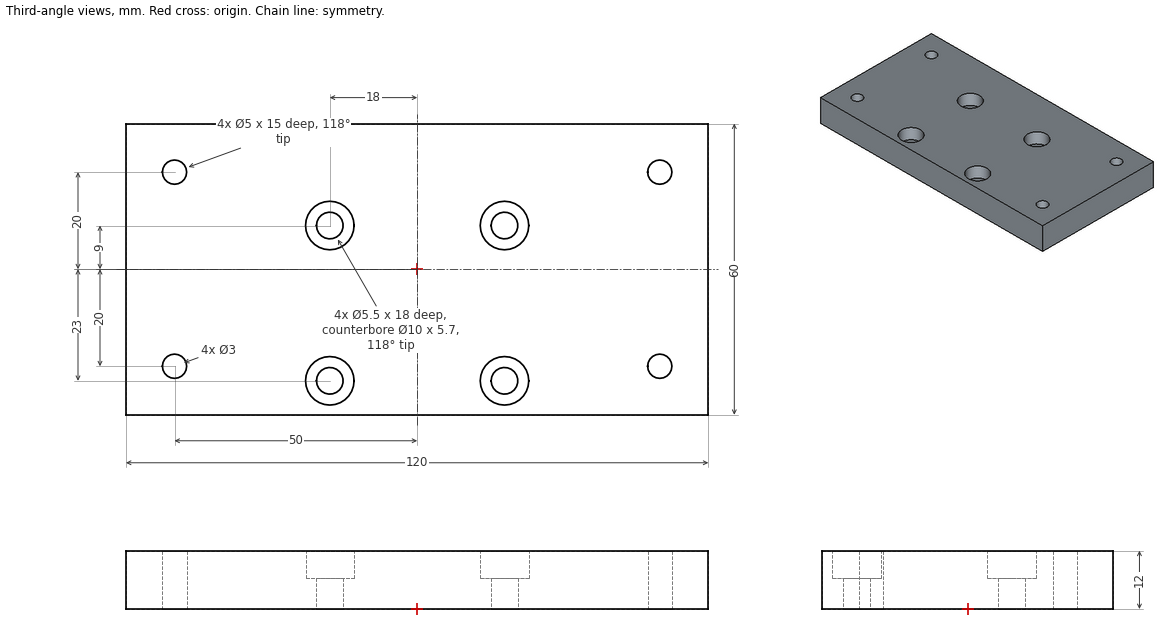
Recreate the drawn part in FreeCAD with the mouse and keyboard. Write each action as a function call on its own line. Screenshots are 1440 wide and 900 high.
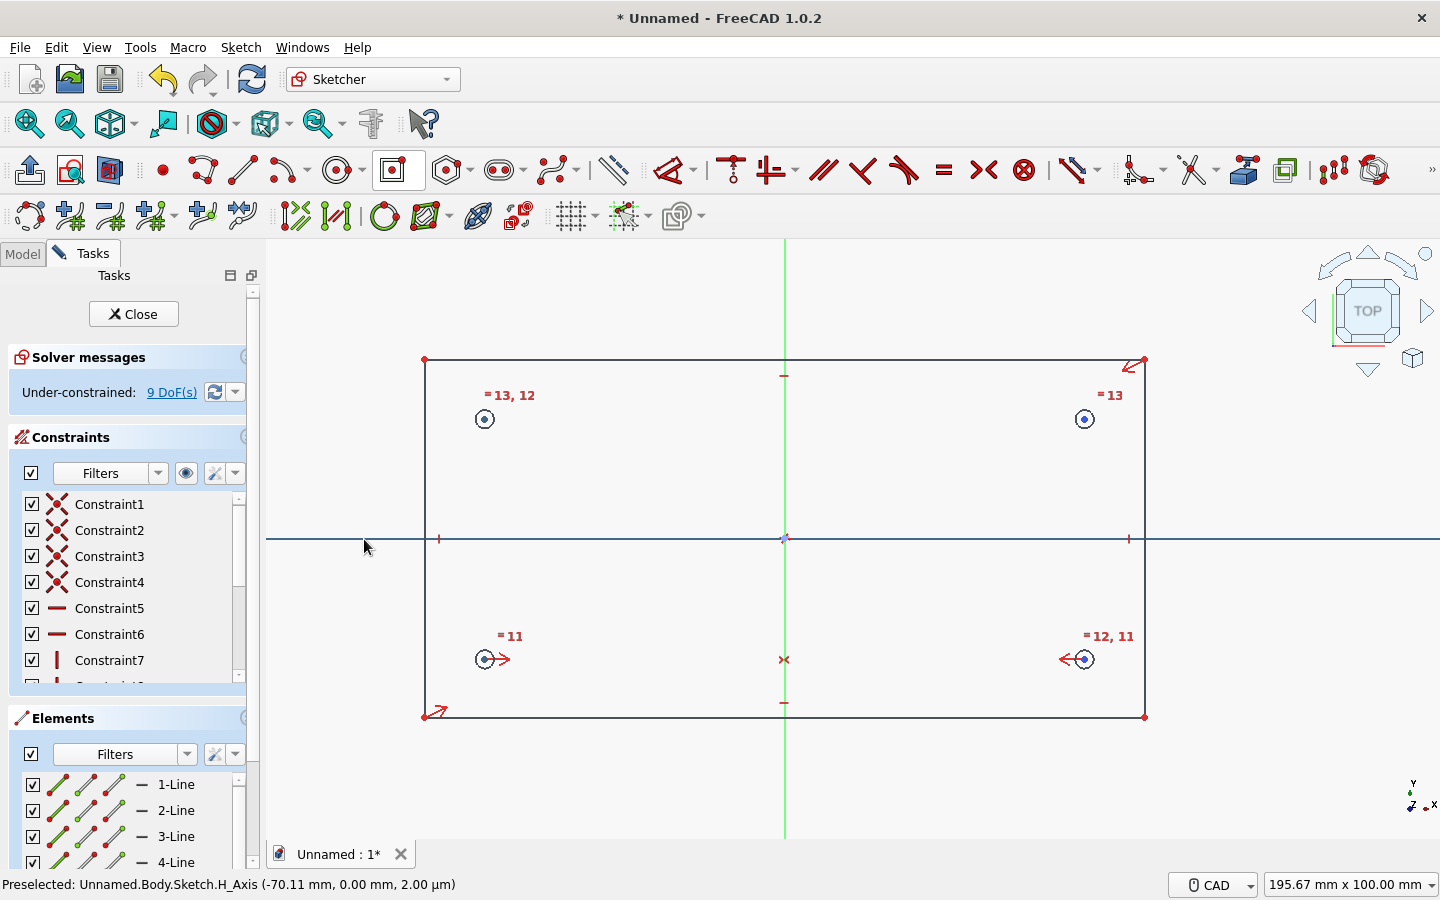
click(984, 170)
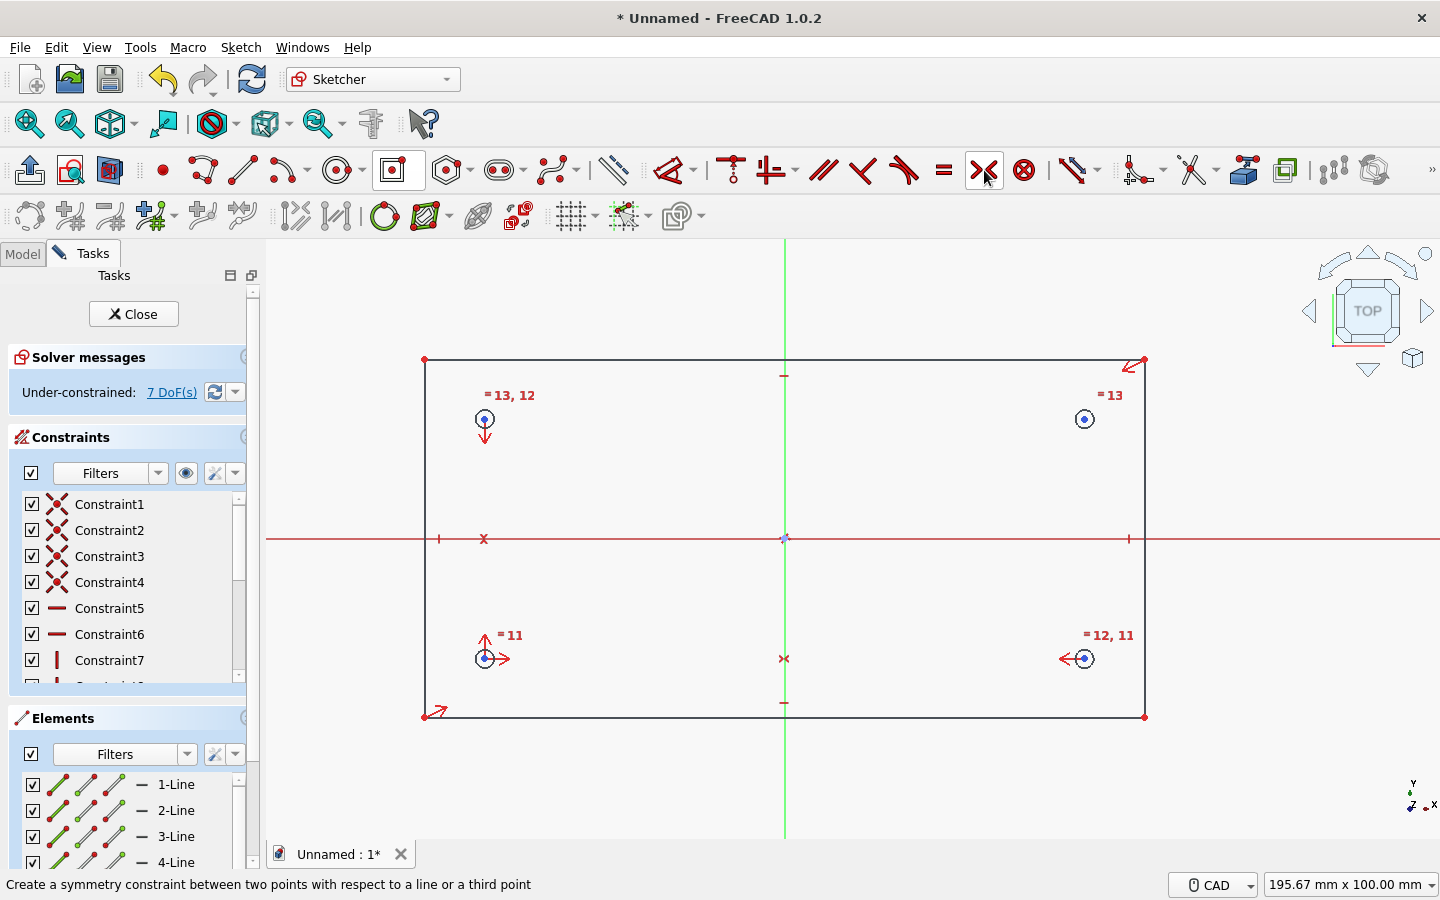
click(1085, 659)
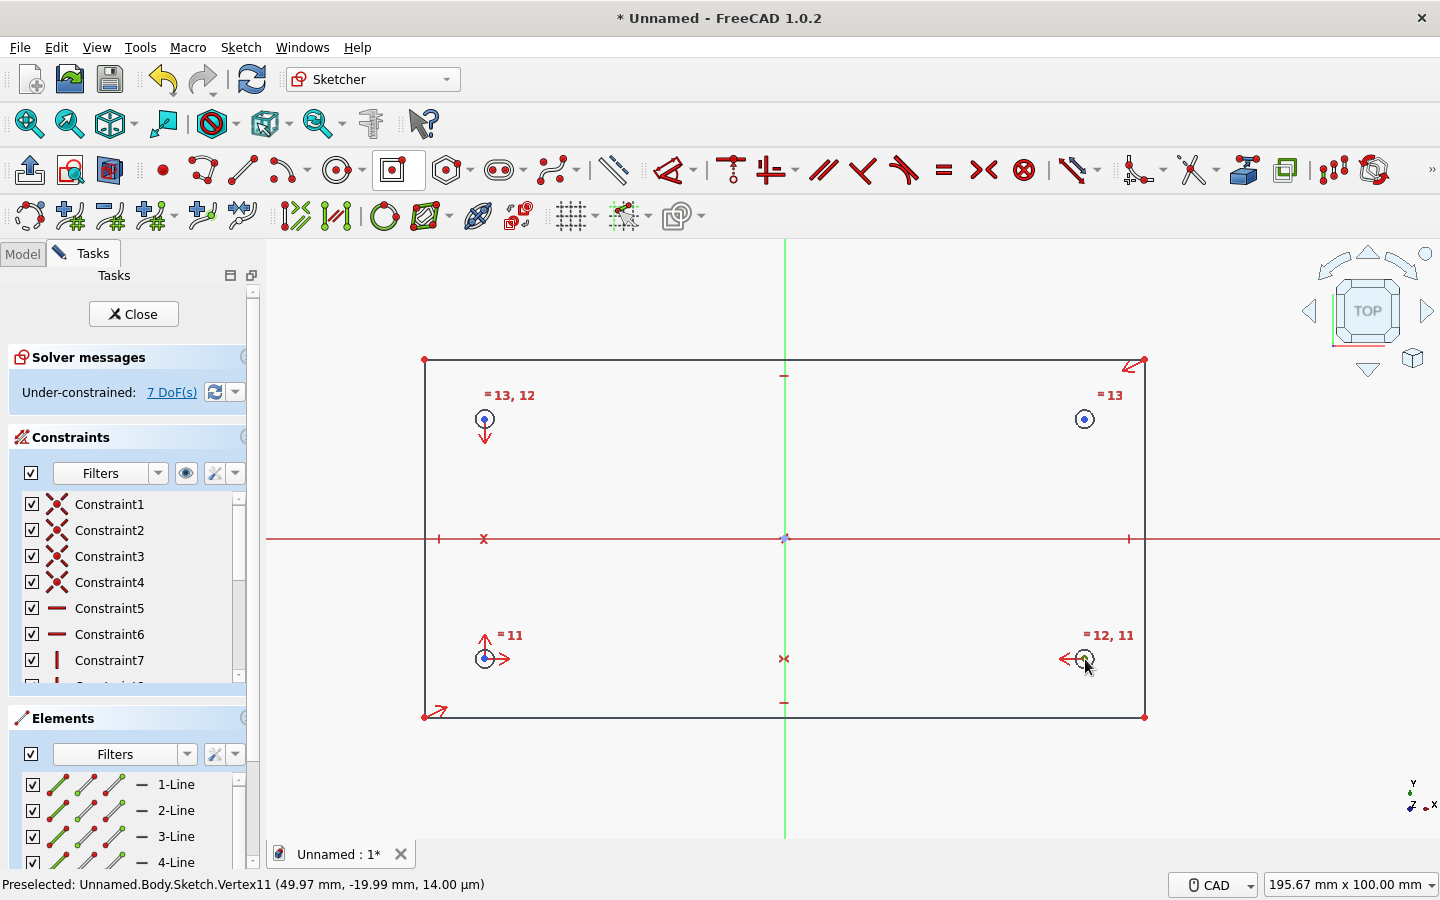
click(1085, 419)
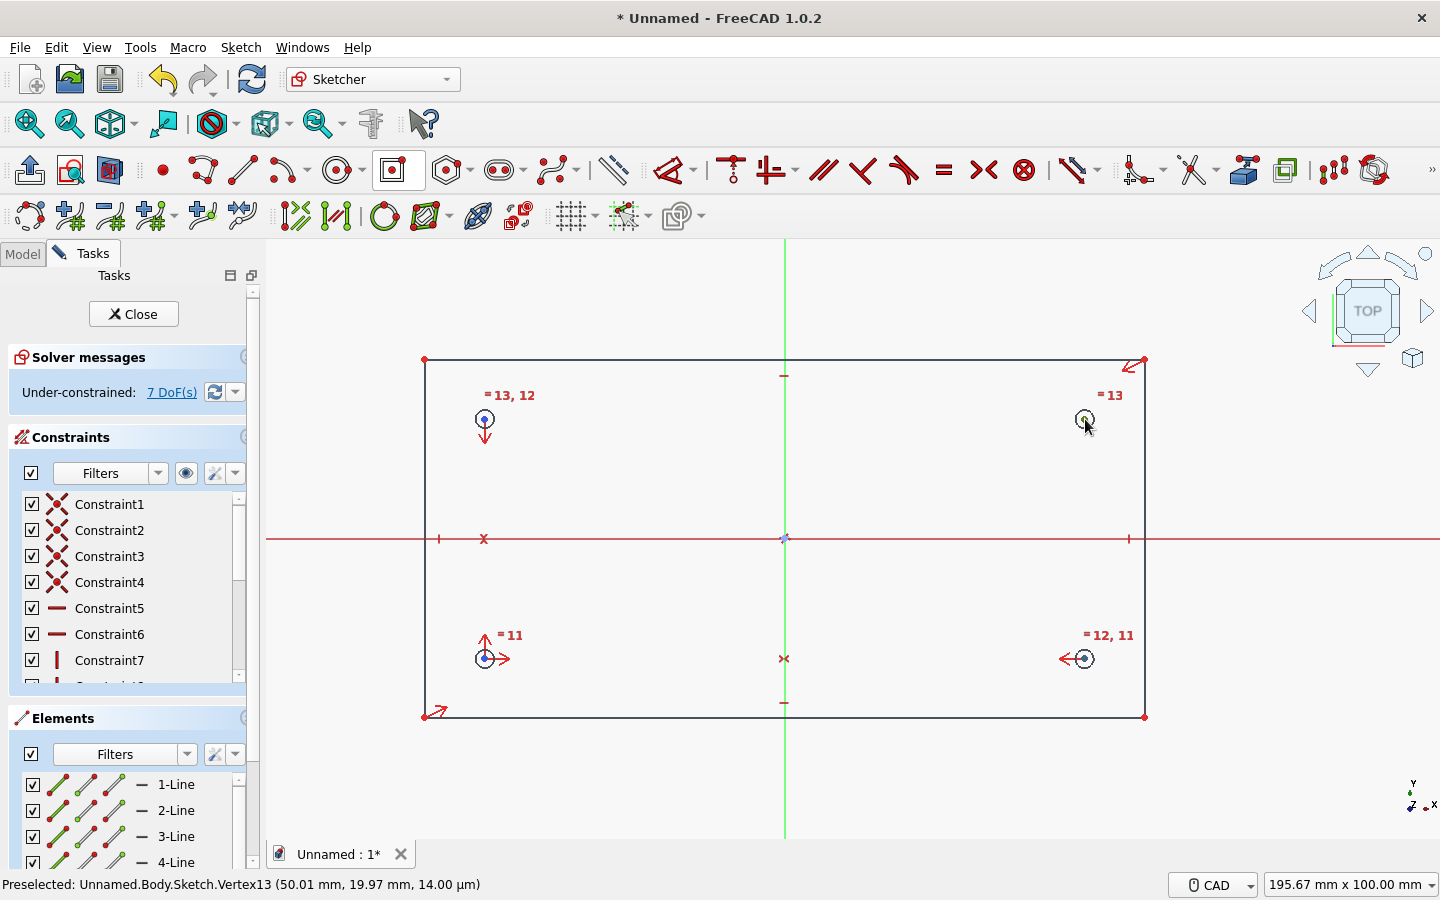
click(364, 539)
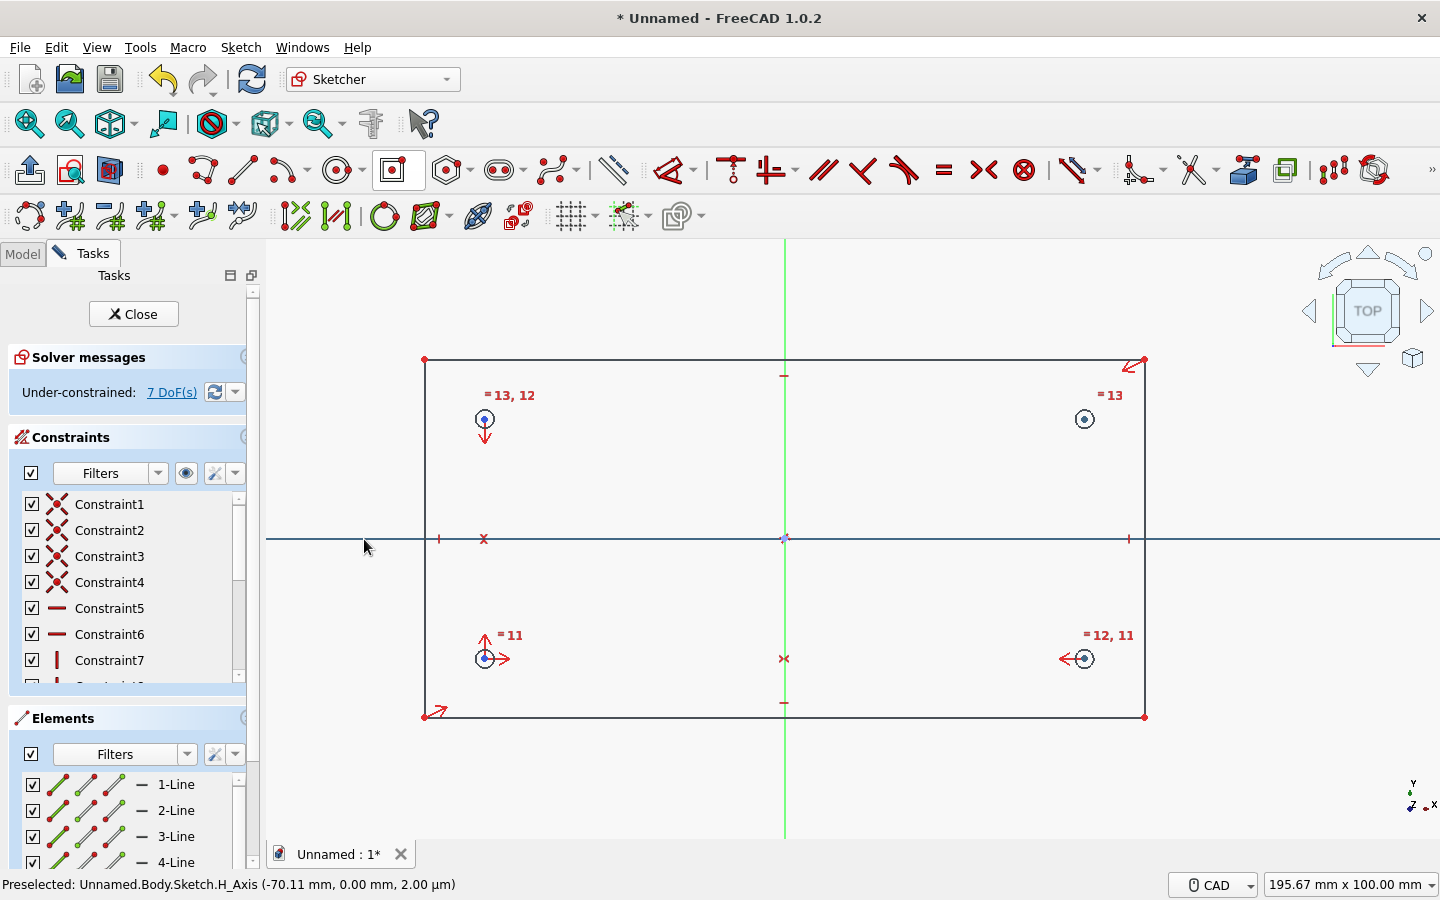
click(984, 170)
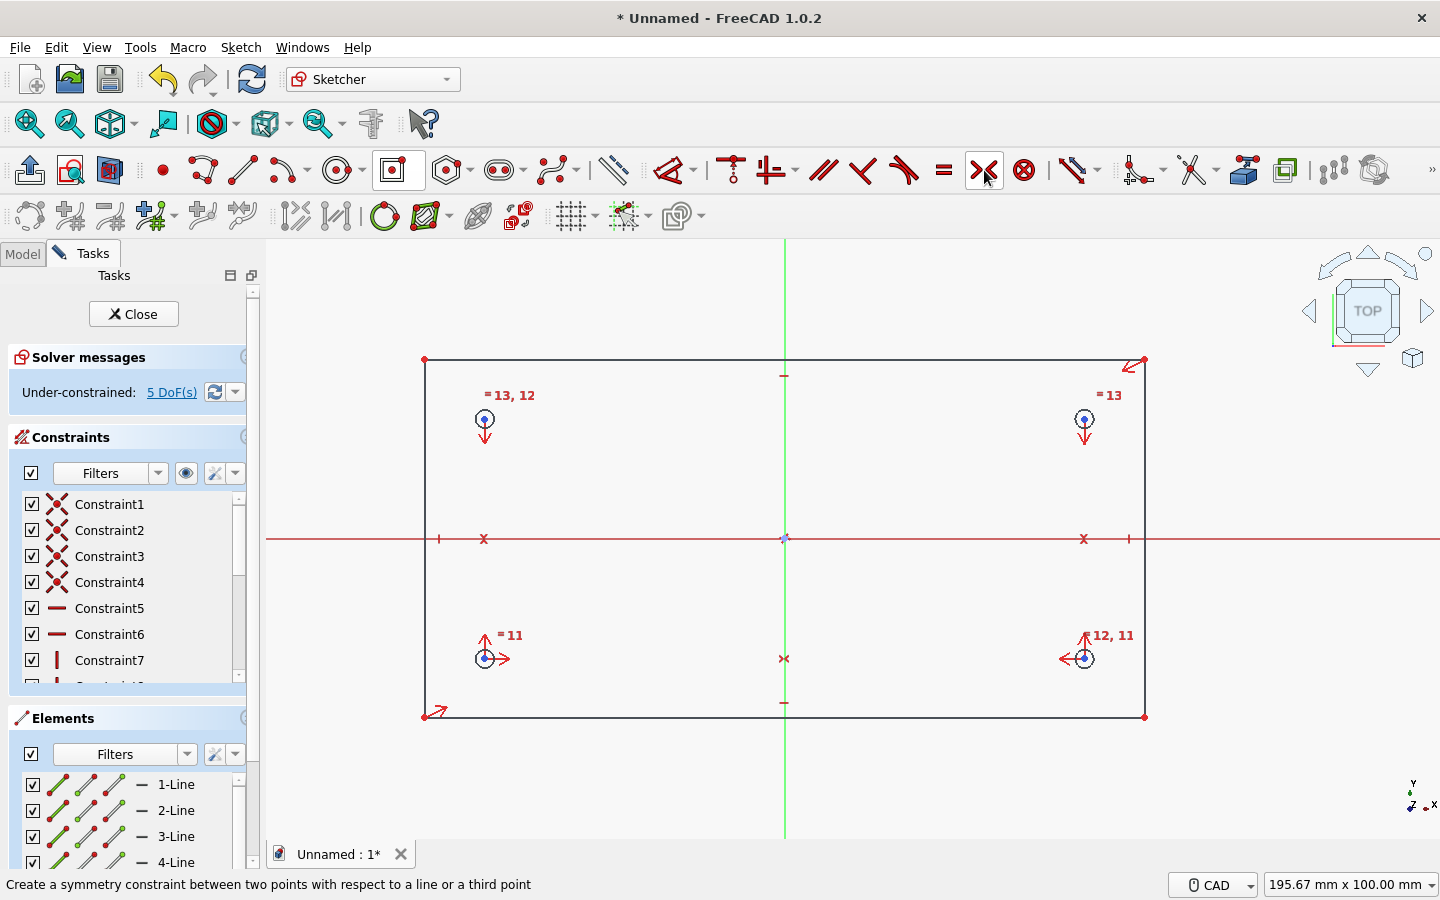
click(668, 170)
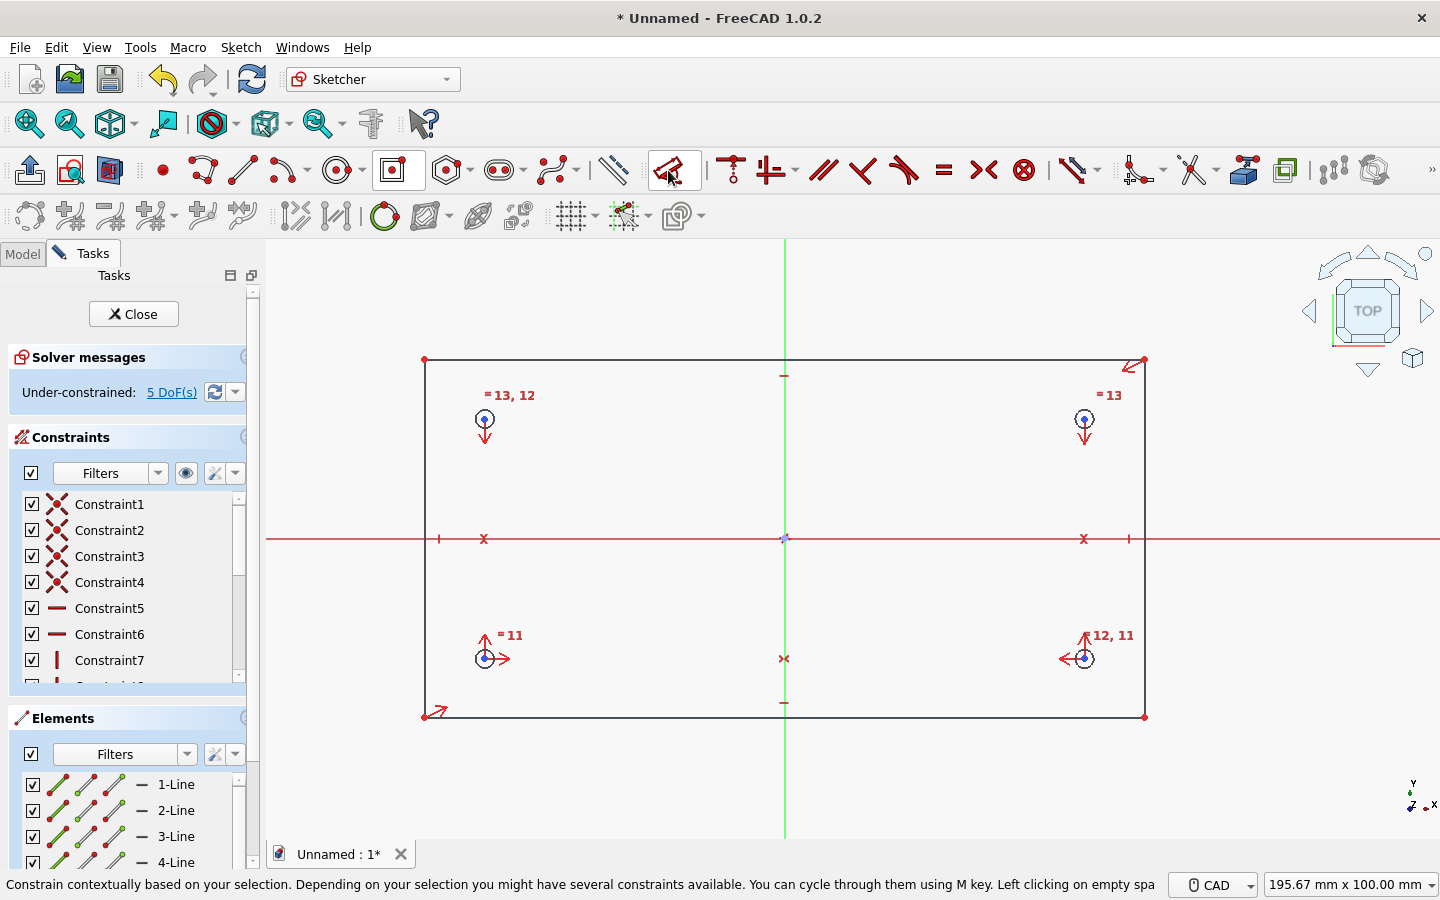
scroll(491, 653, up, 4)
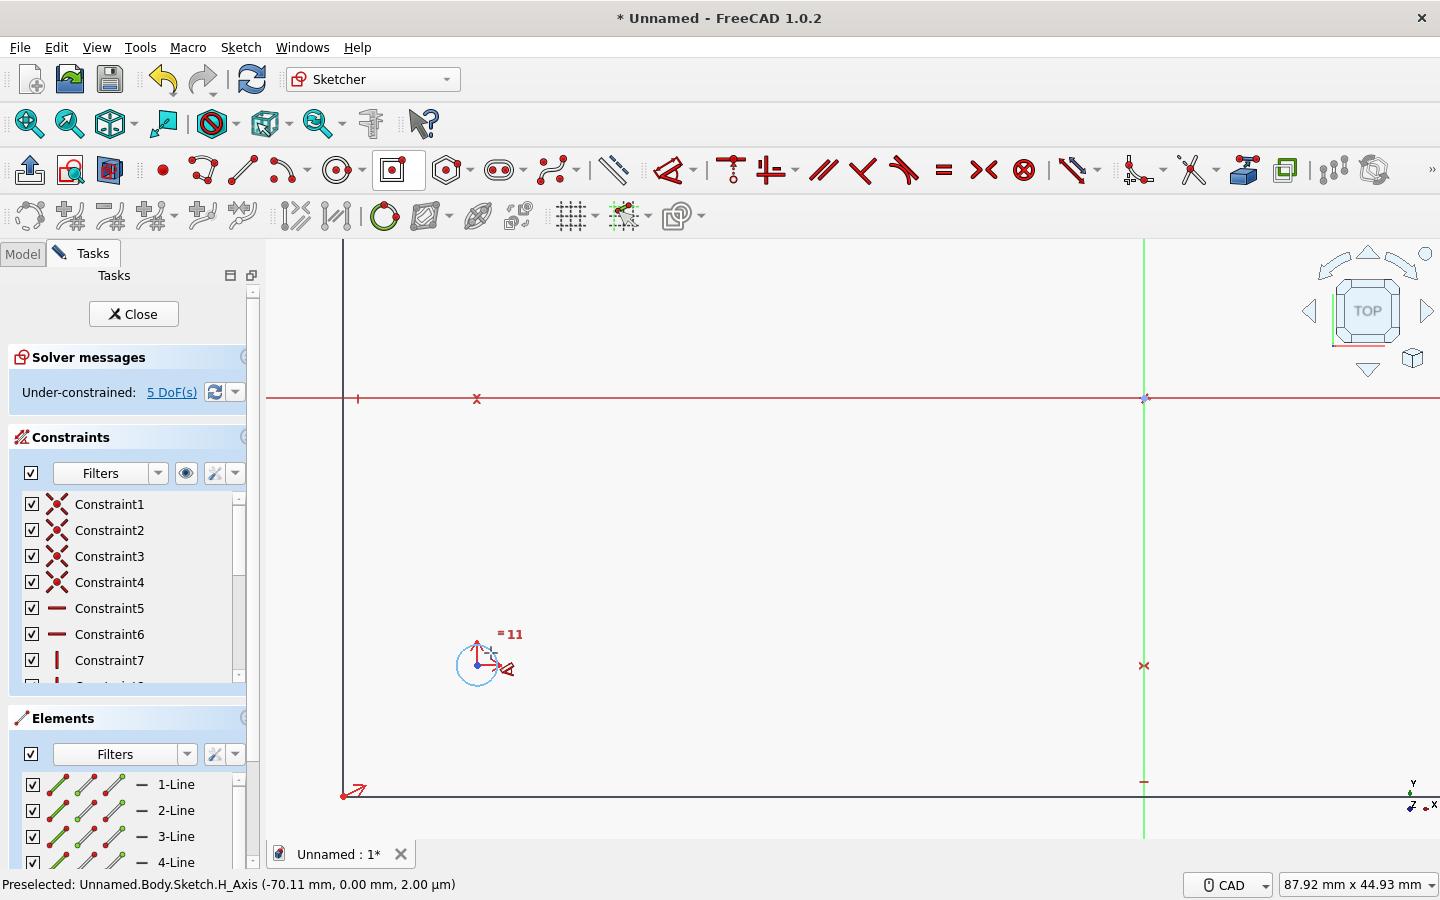
click(491, 651)
click(513, 628)